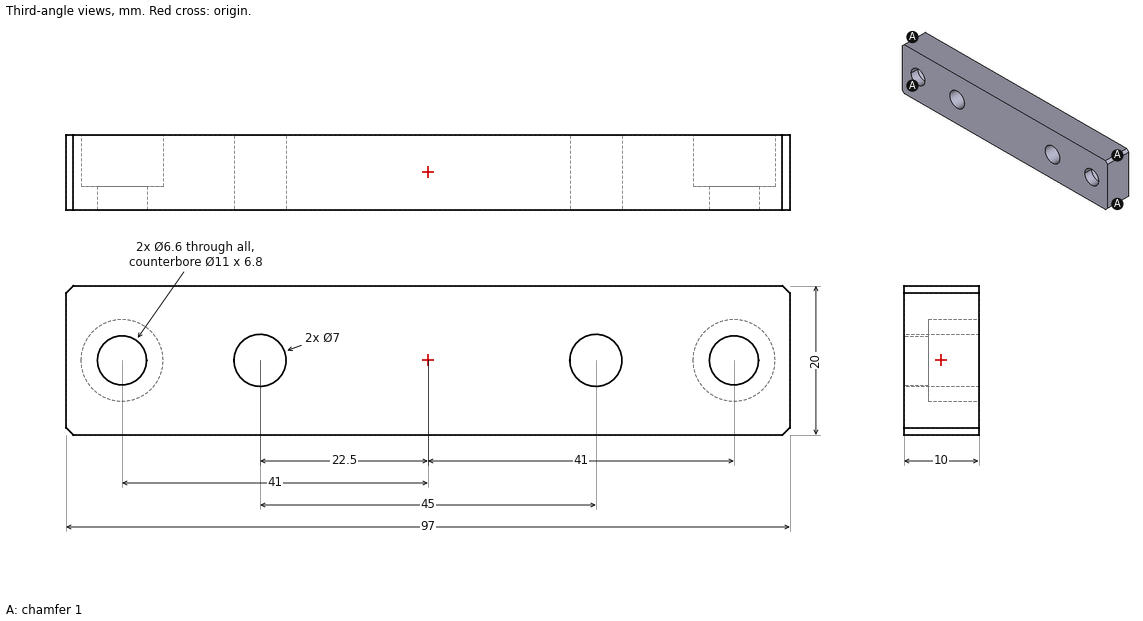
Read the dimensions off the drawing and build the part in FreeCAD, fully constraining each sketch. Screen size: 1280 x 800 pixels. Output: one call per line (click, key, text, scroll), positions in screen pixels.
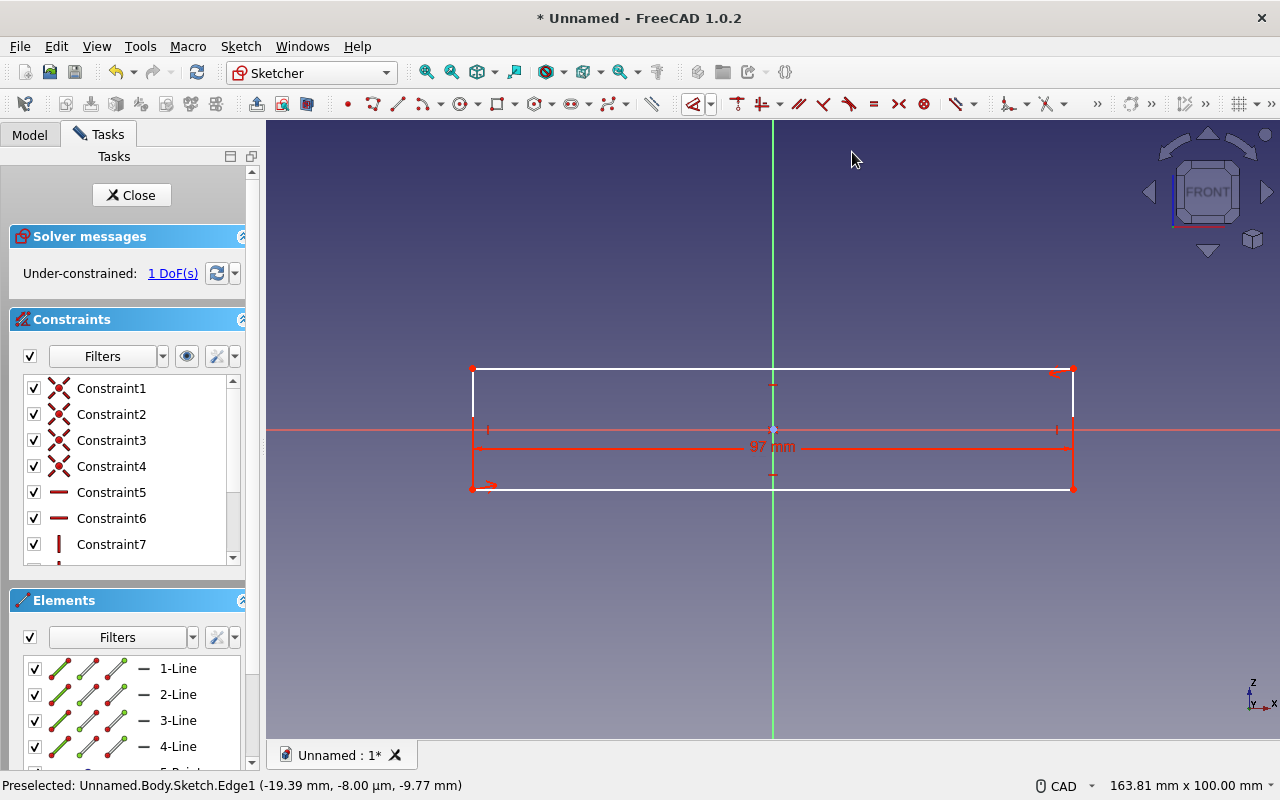
click(1073, 454)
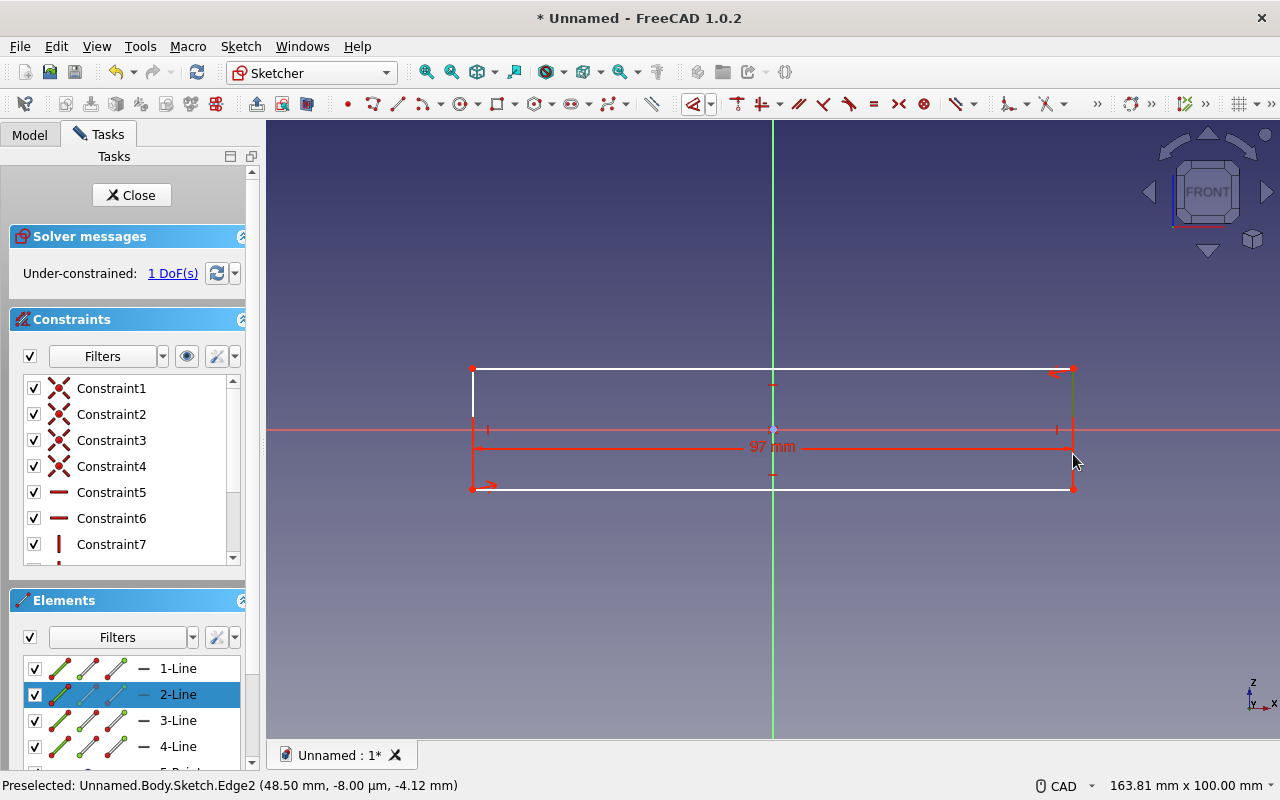
key(i)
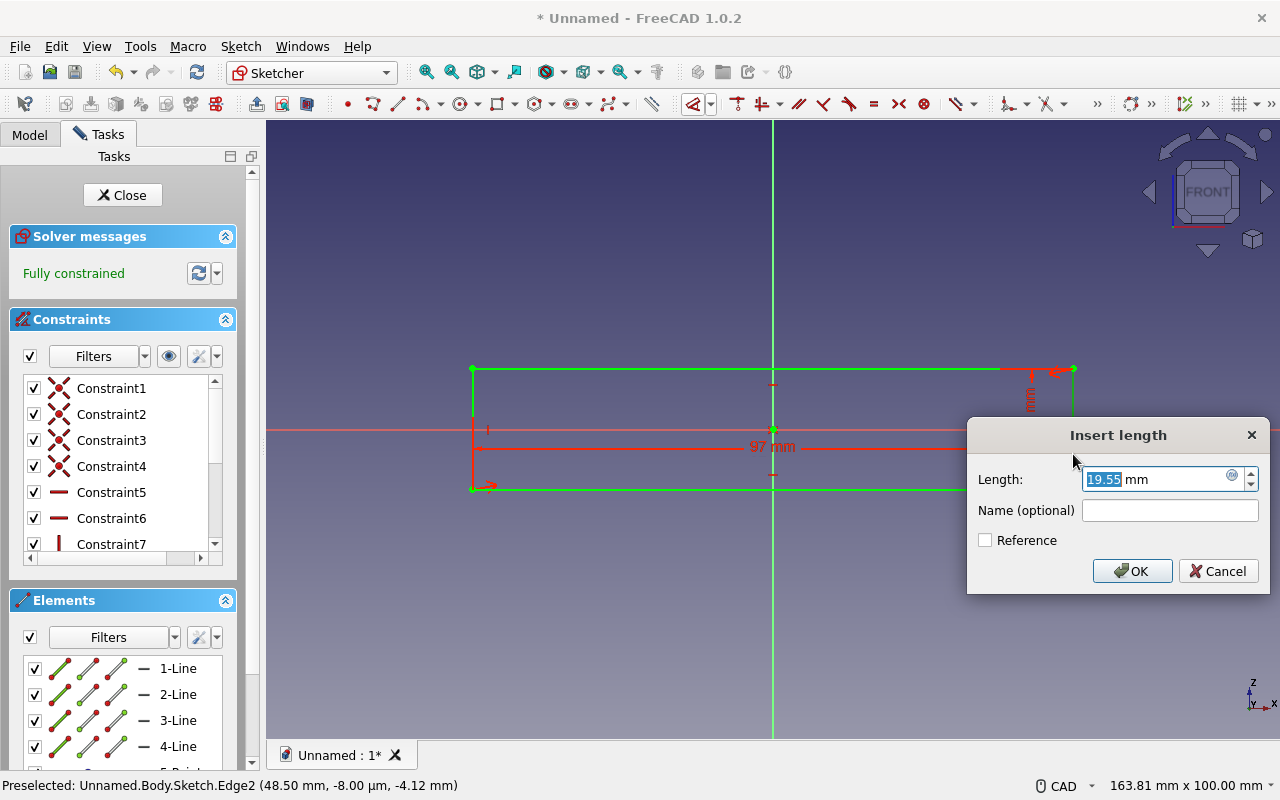
text(20)
key(Return)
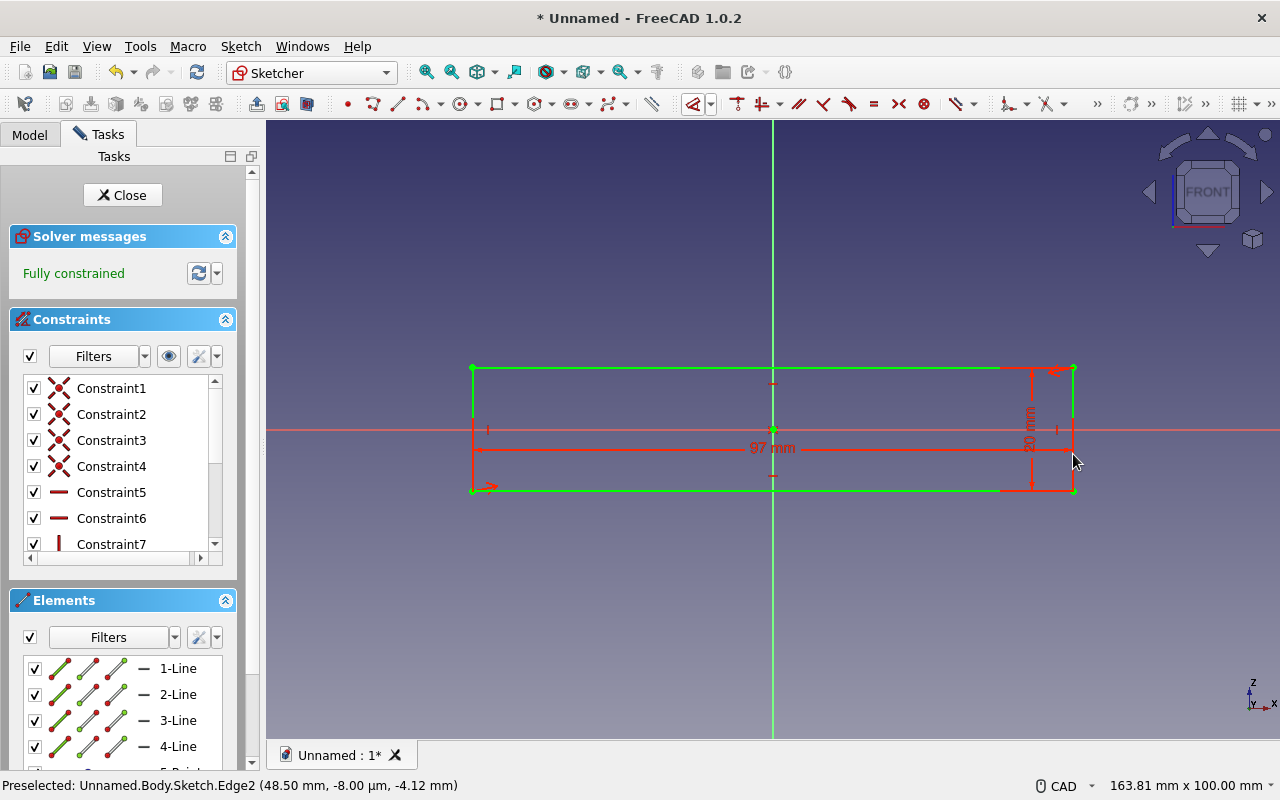
click(123, 195)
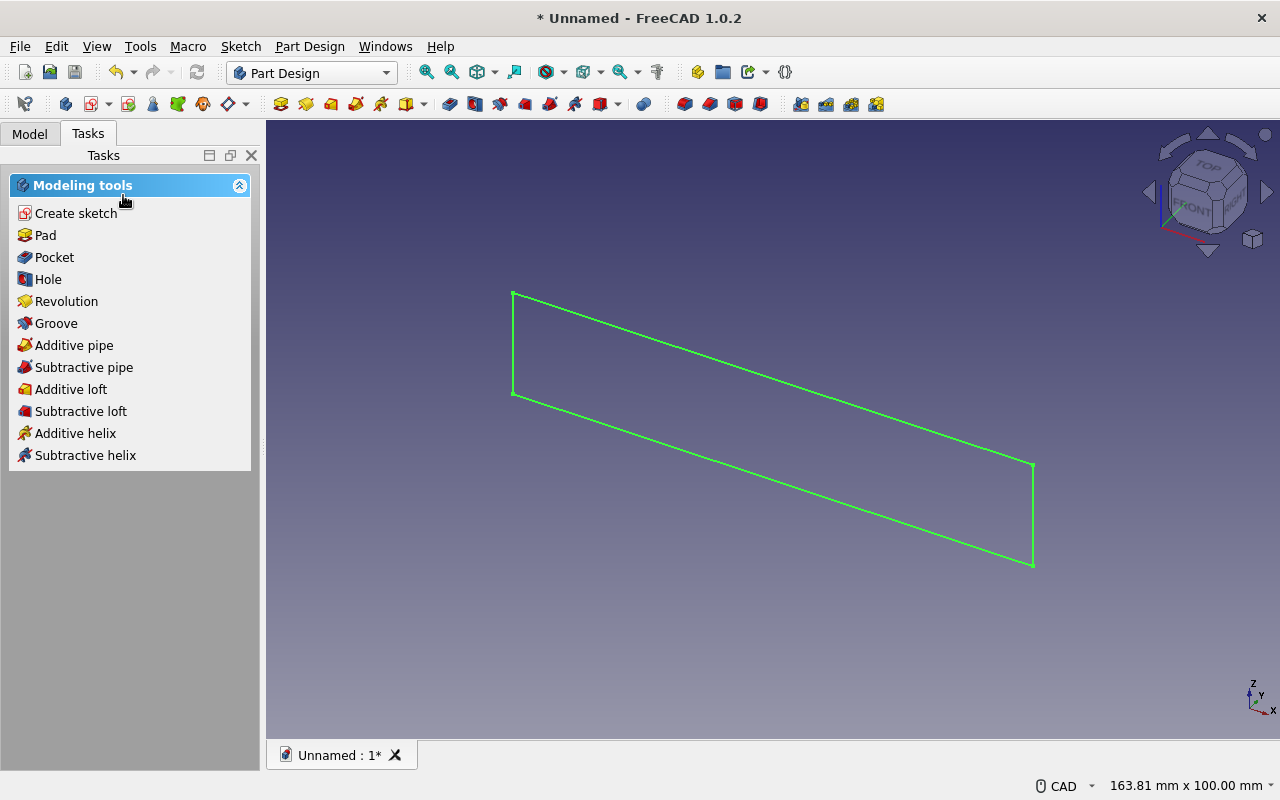
click(281, 104)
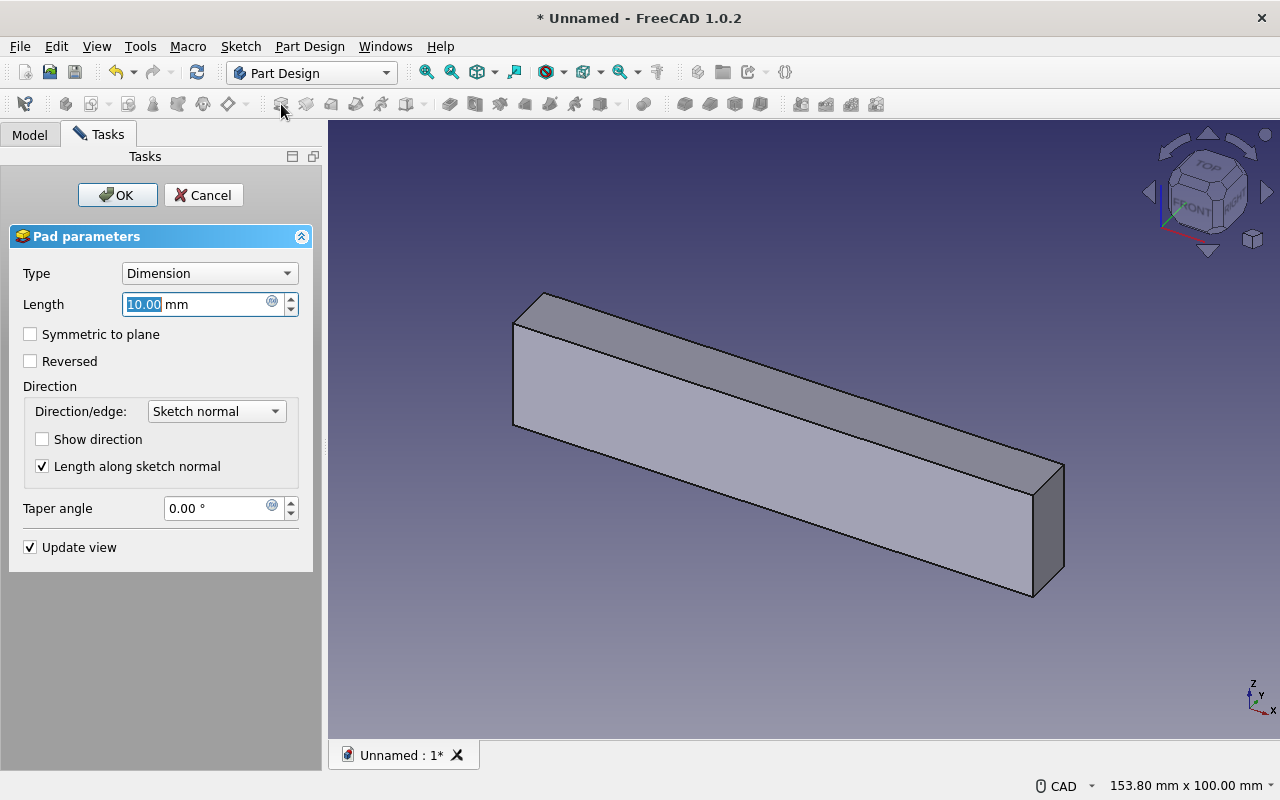
text(10)
key(Tab)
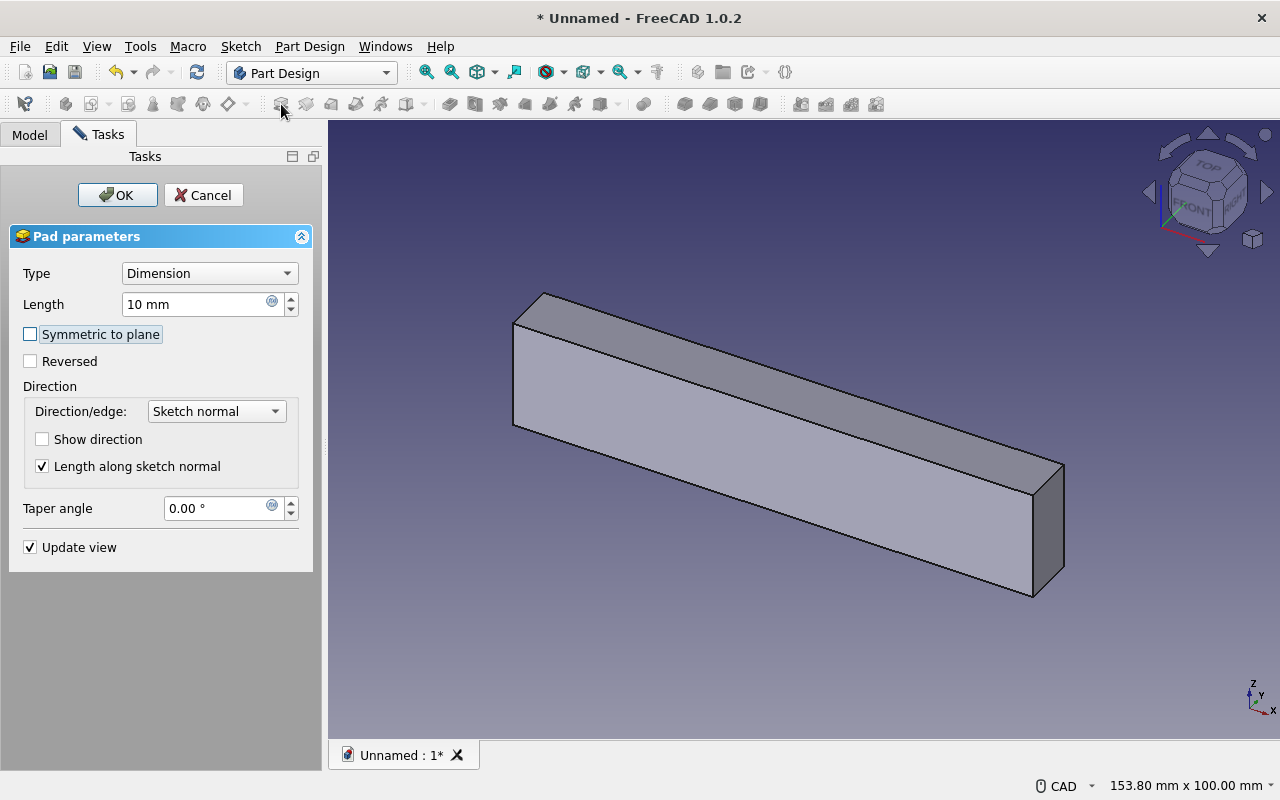
click(31, 334)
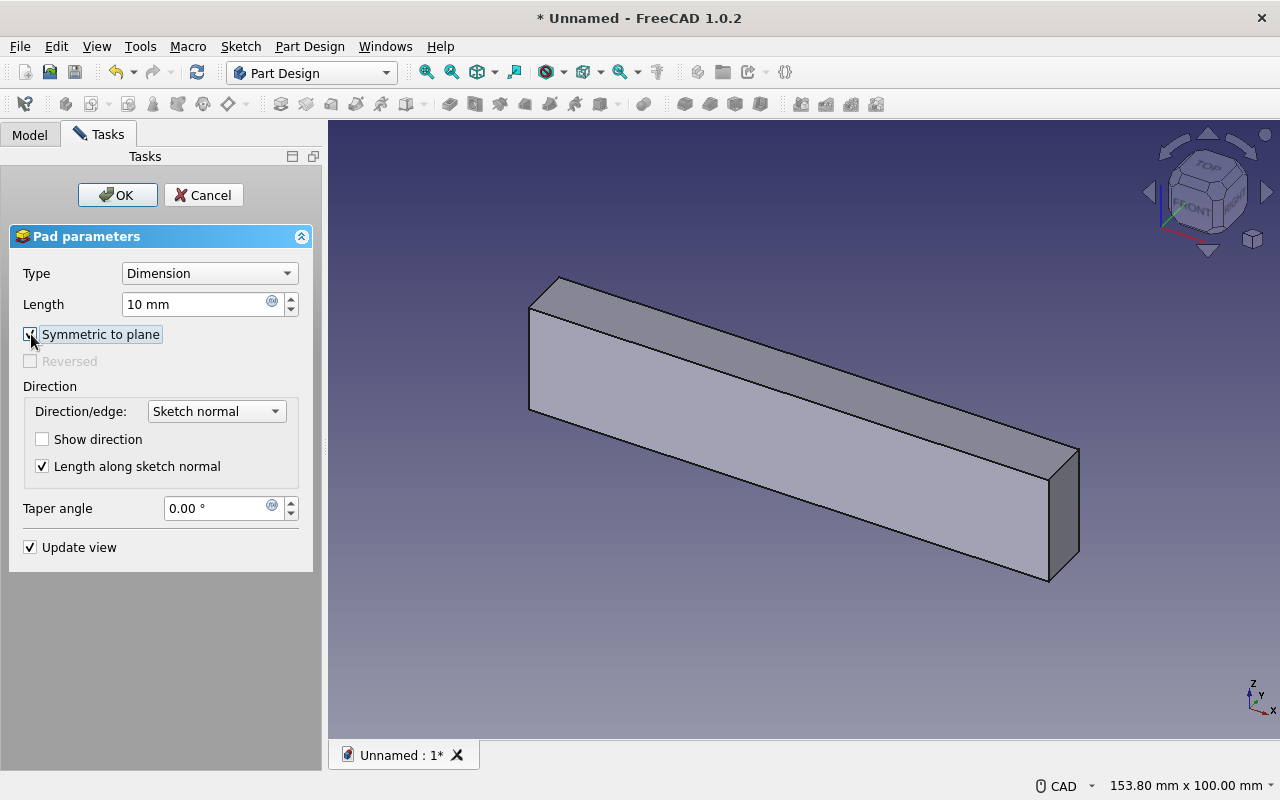
click(118, 195)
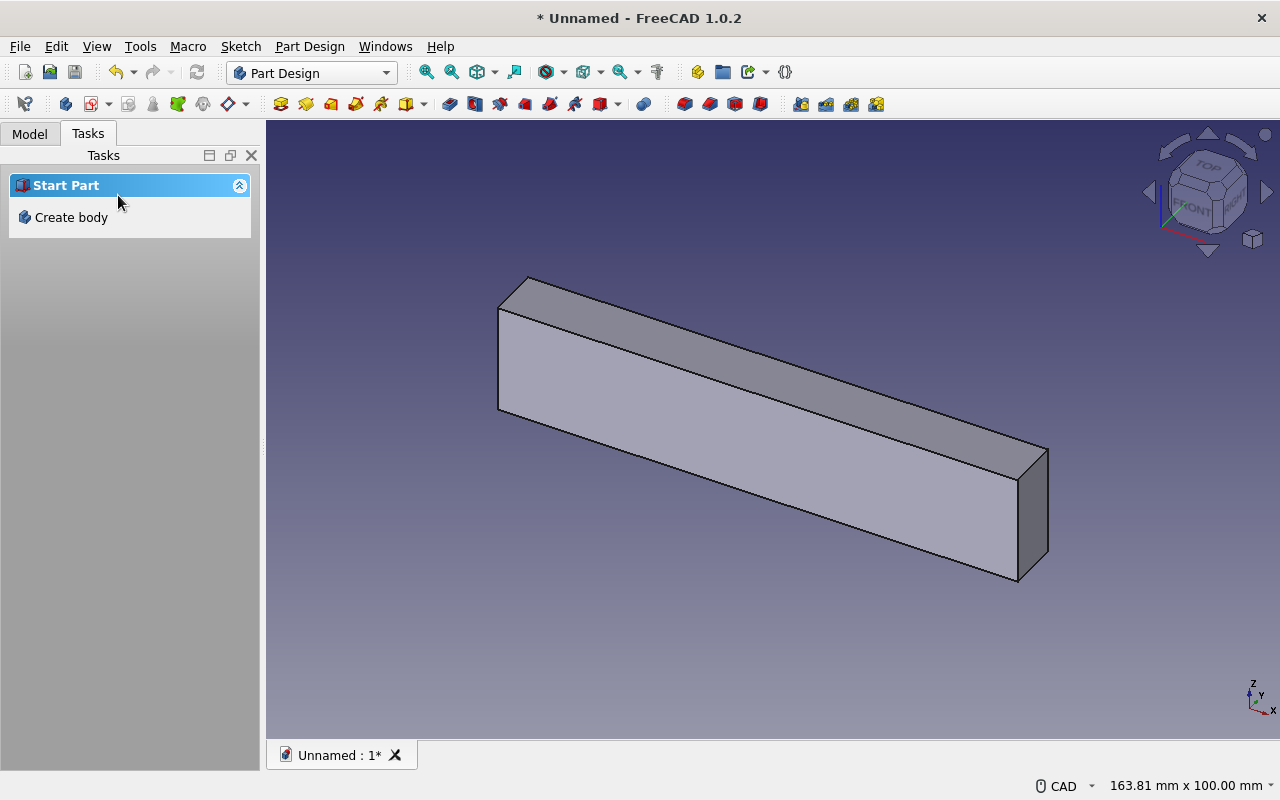
key(4)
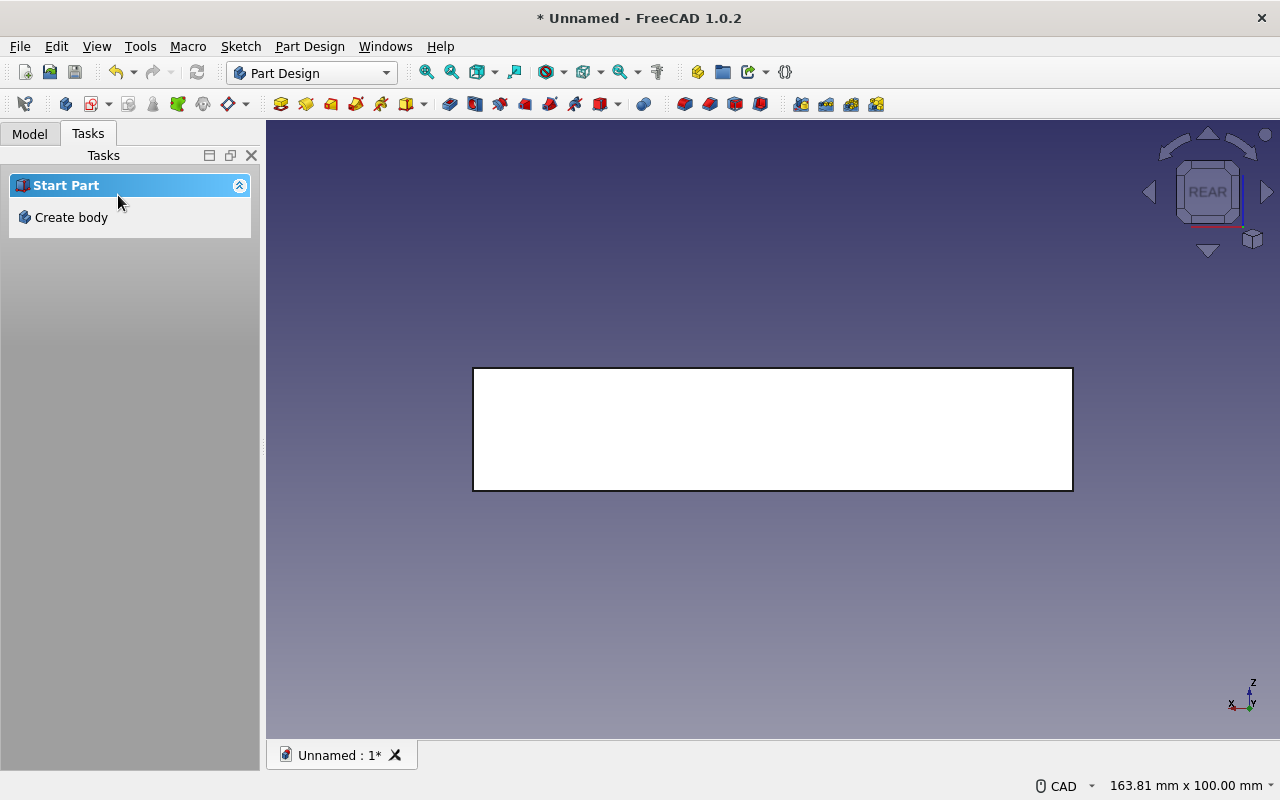
click(601, 428)